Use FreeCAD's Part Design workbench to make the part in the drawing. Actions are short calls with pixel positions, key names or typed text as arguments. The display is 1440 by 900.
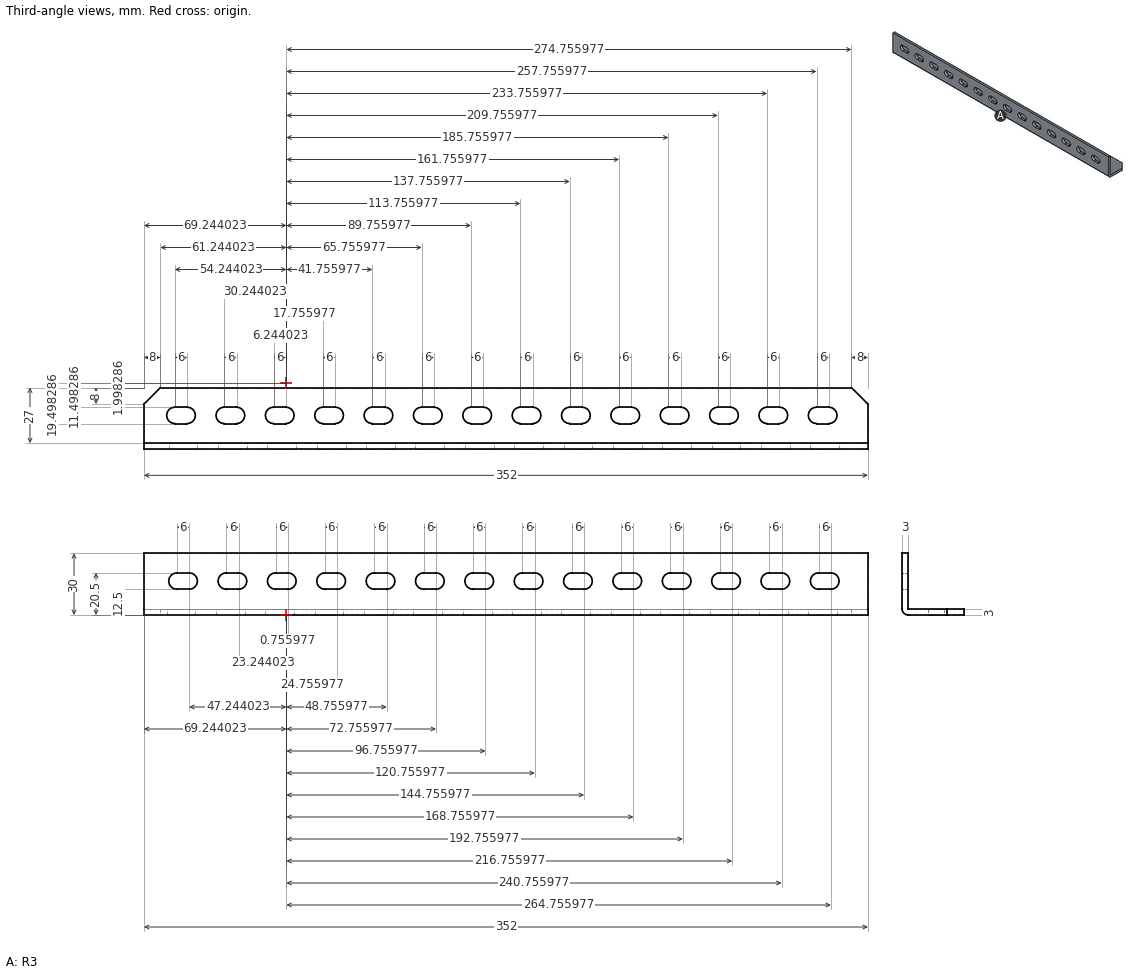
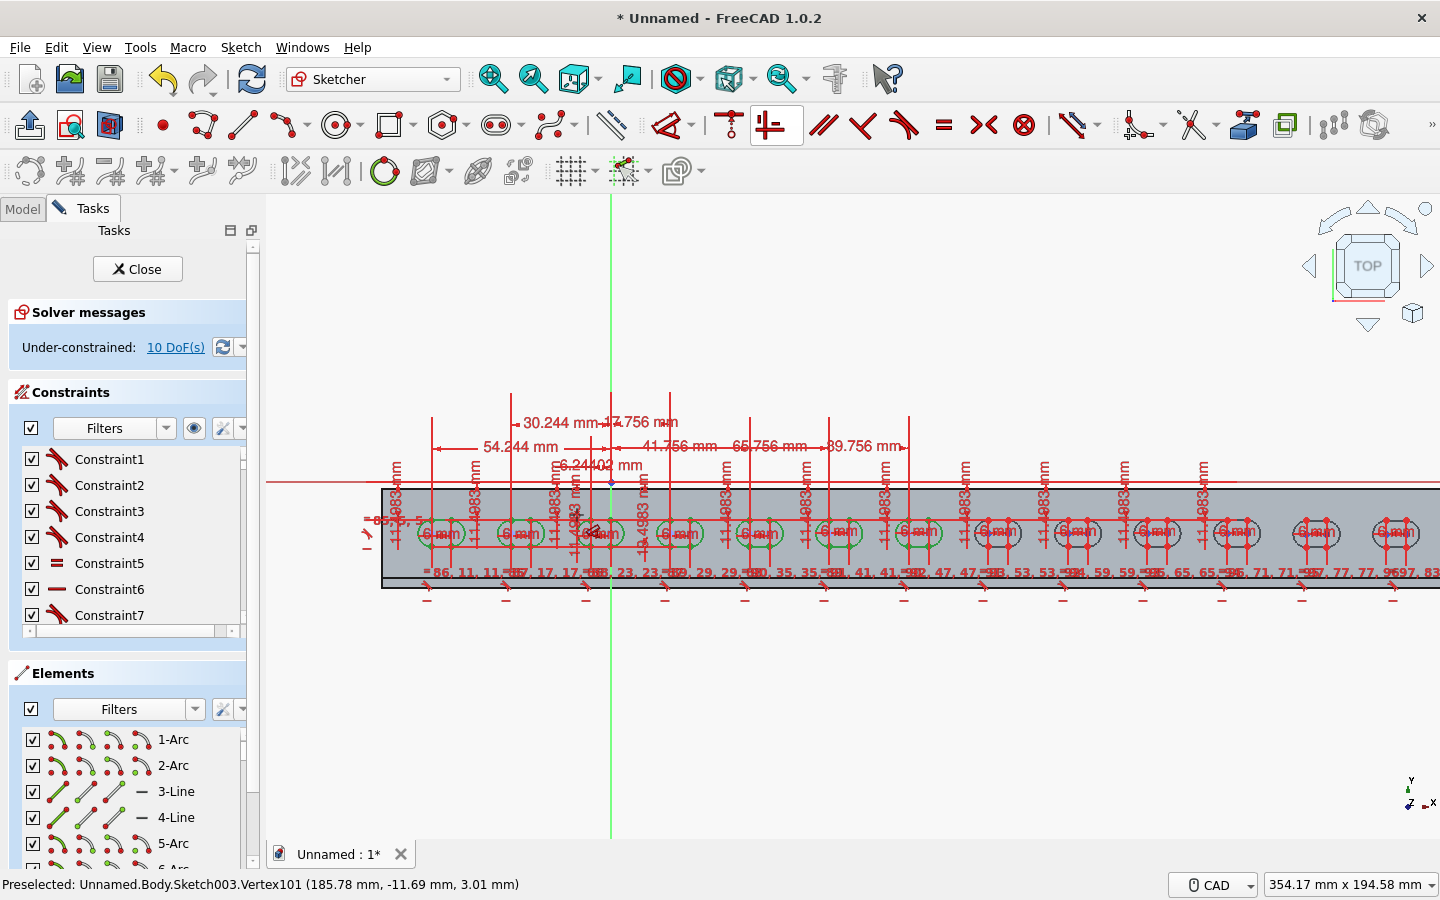
scroll(431, 521, down, 2)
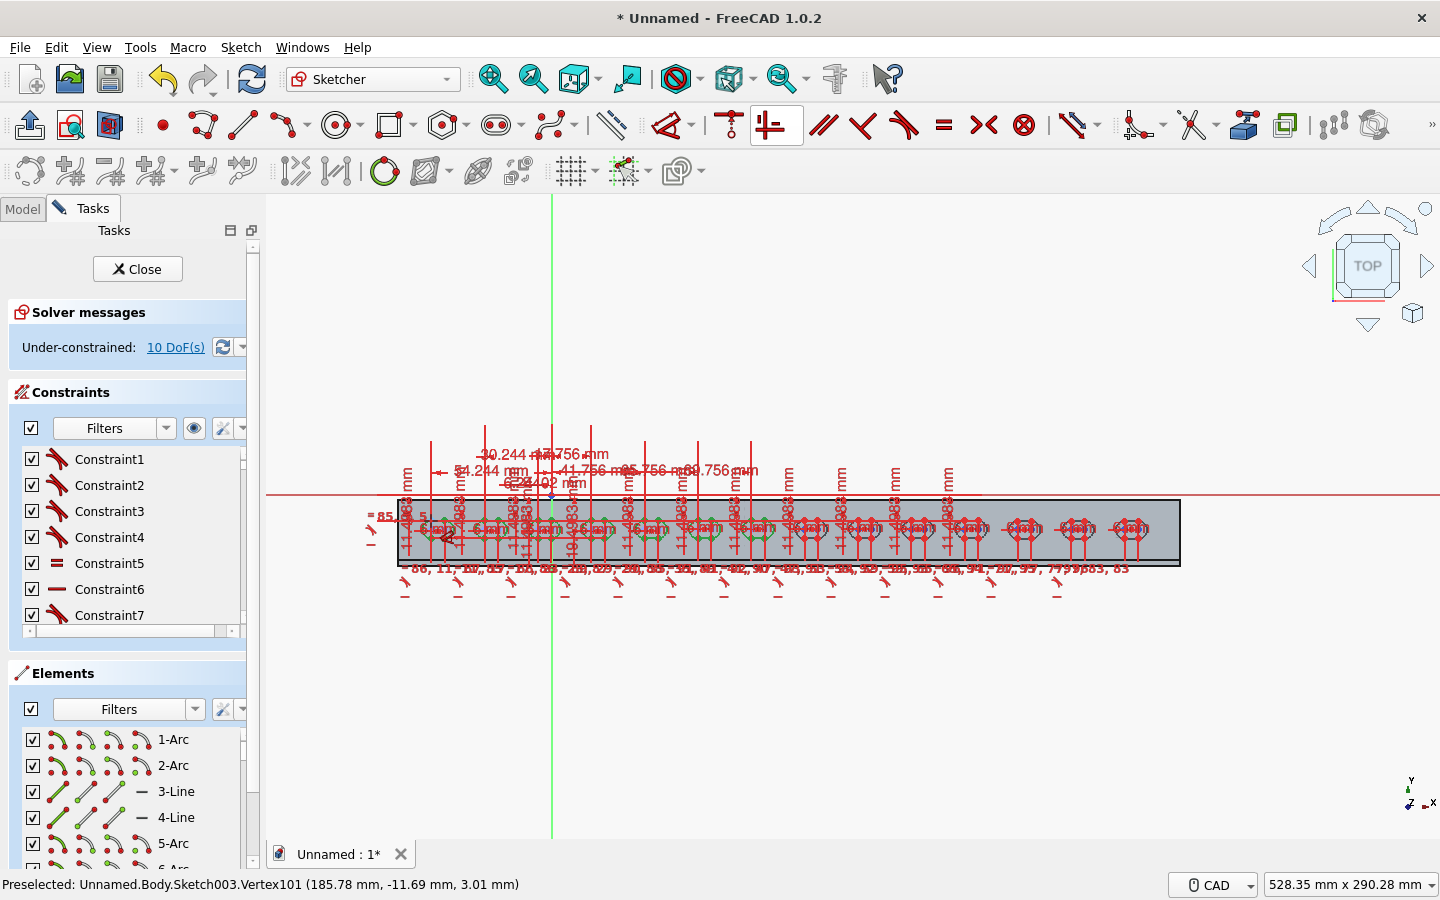
scroll(1018, 521, up, 3)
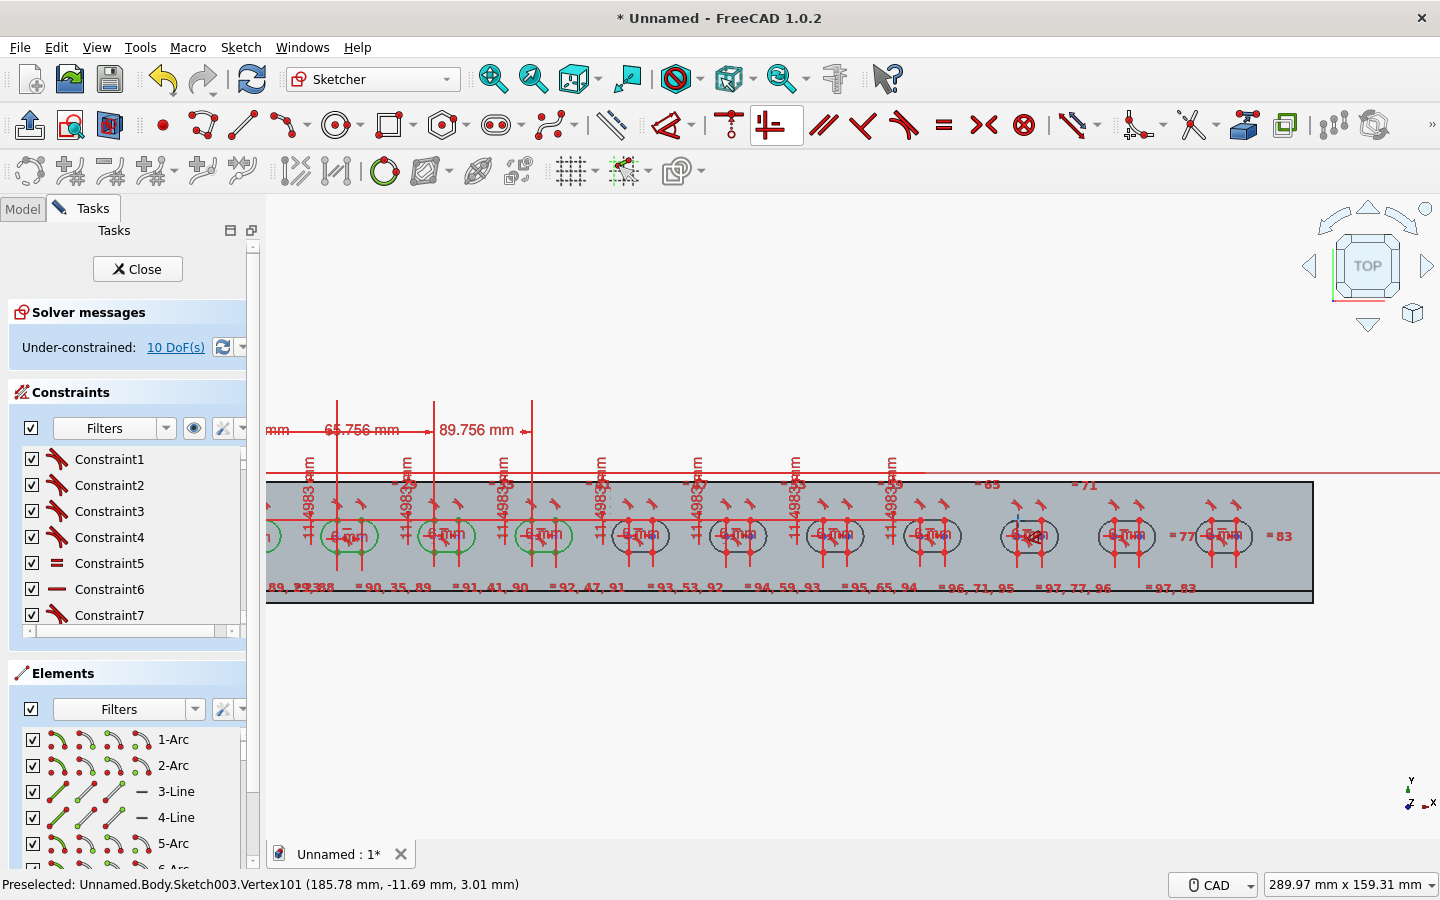
click(1017, 521)
click(1051, 497)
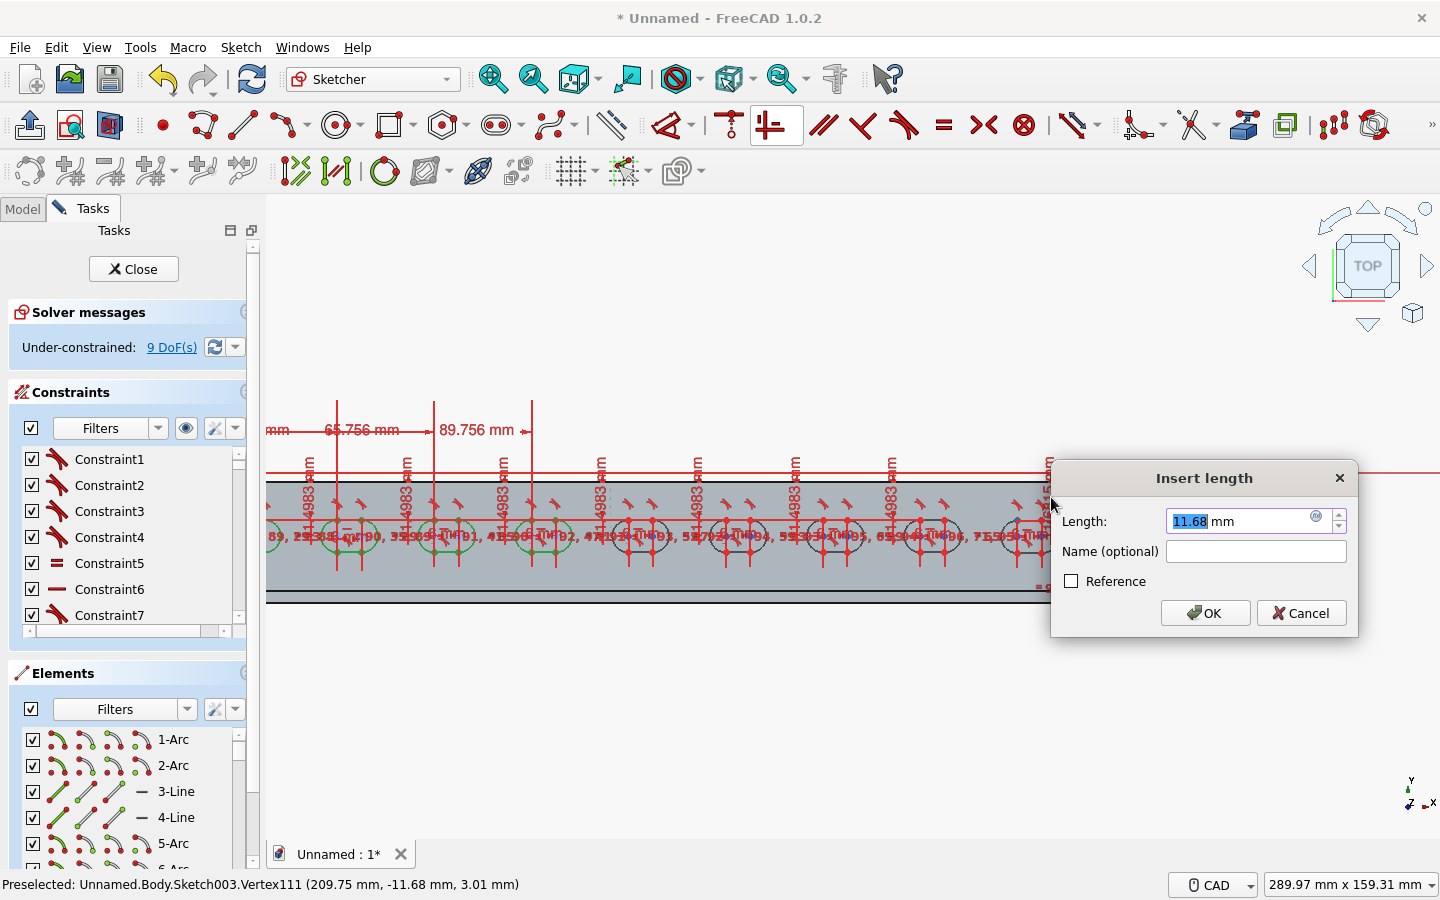
text(11.498286)
key(Return)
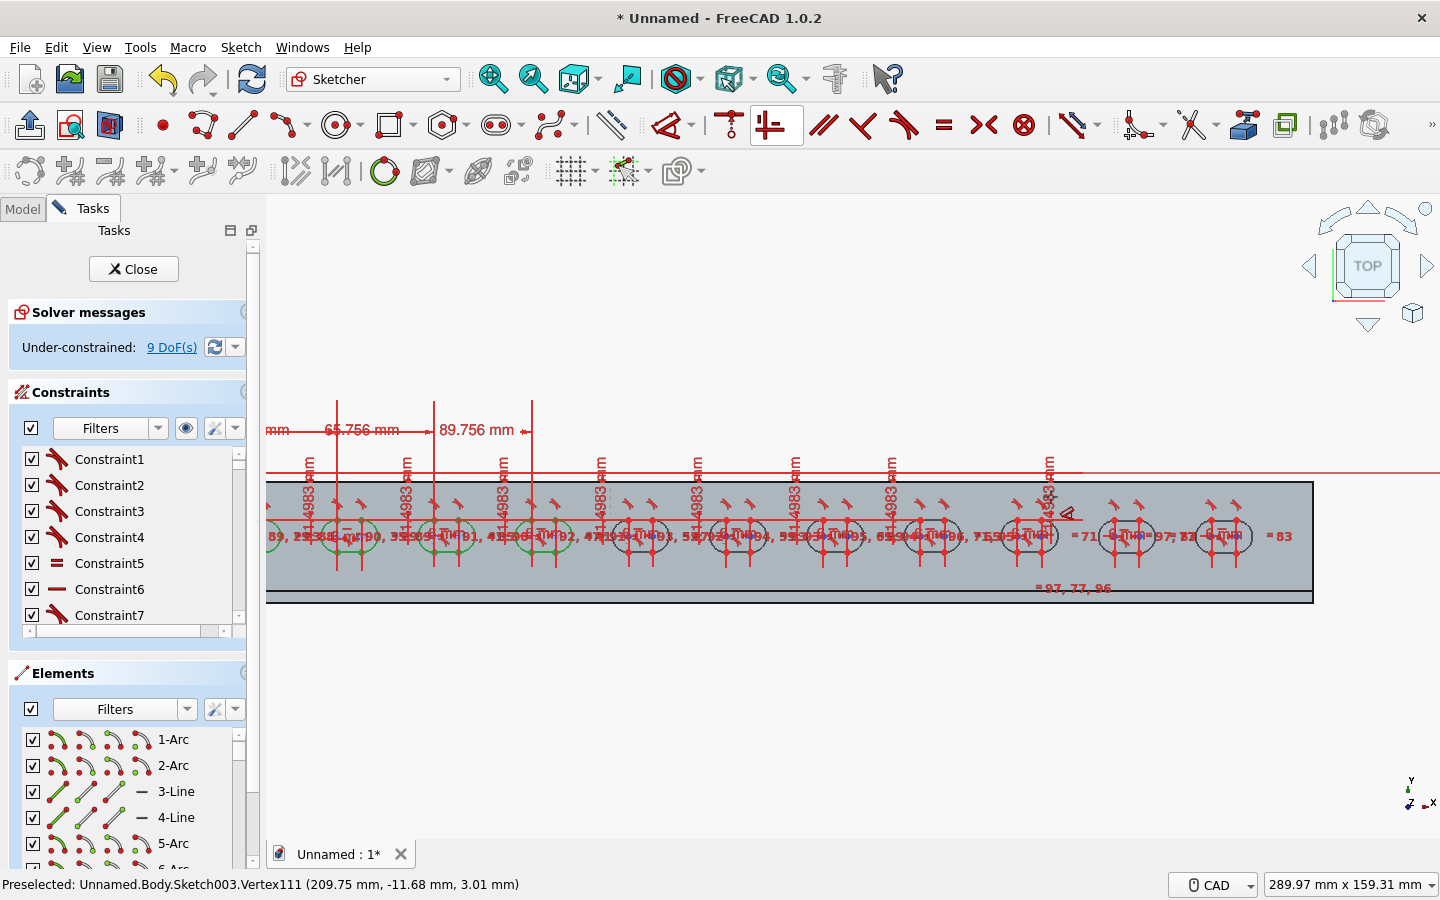
click(1115, 521)
click(1149, 497)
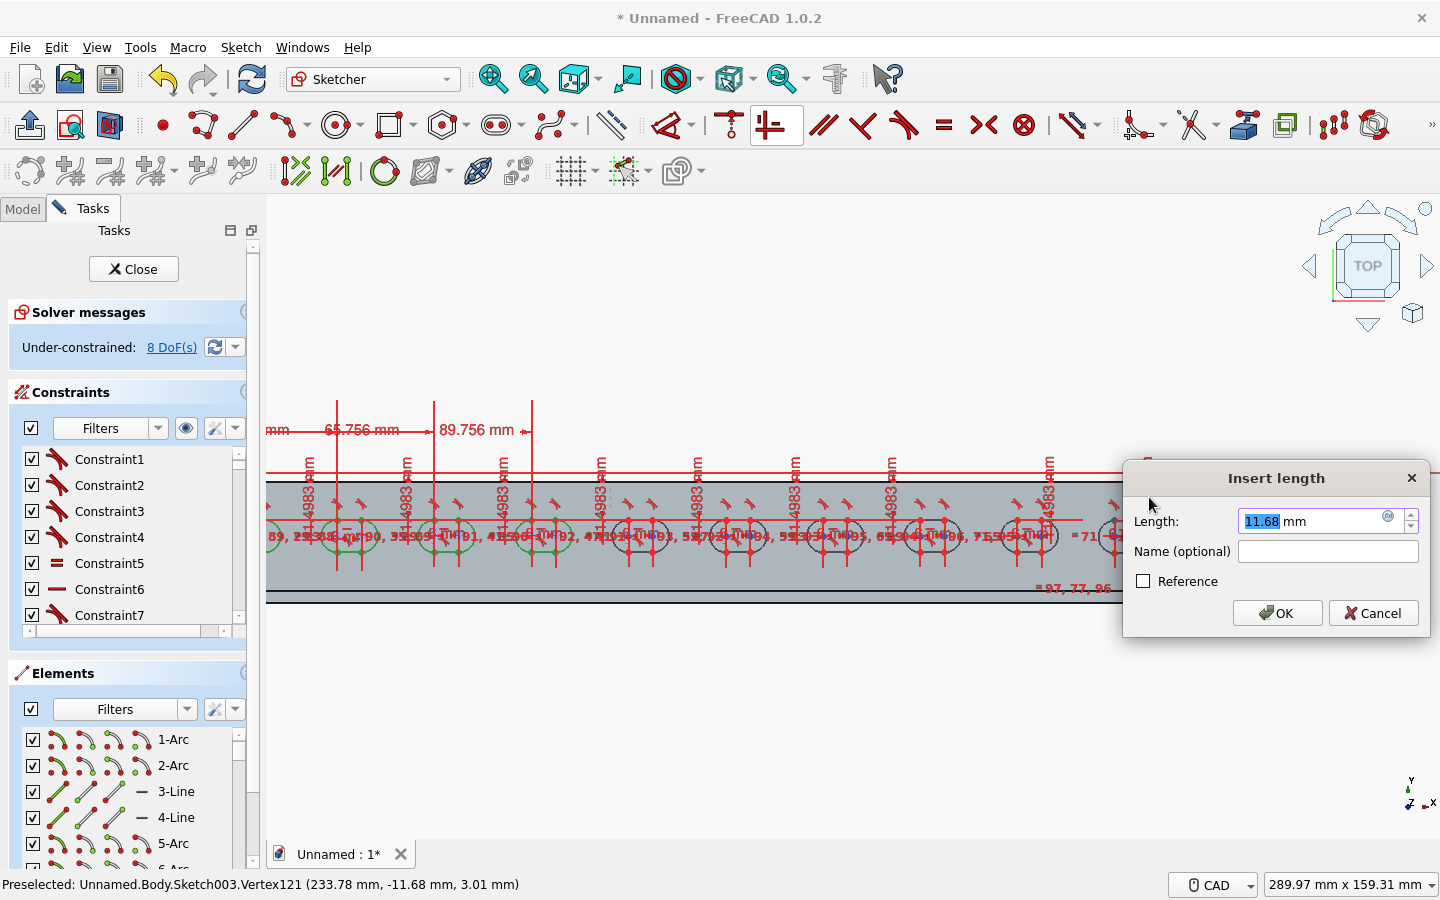
text(11.498286)
key(Return)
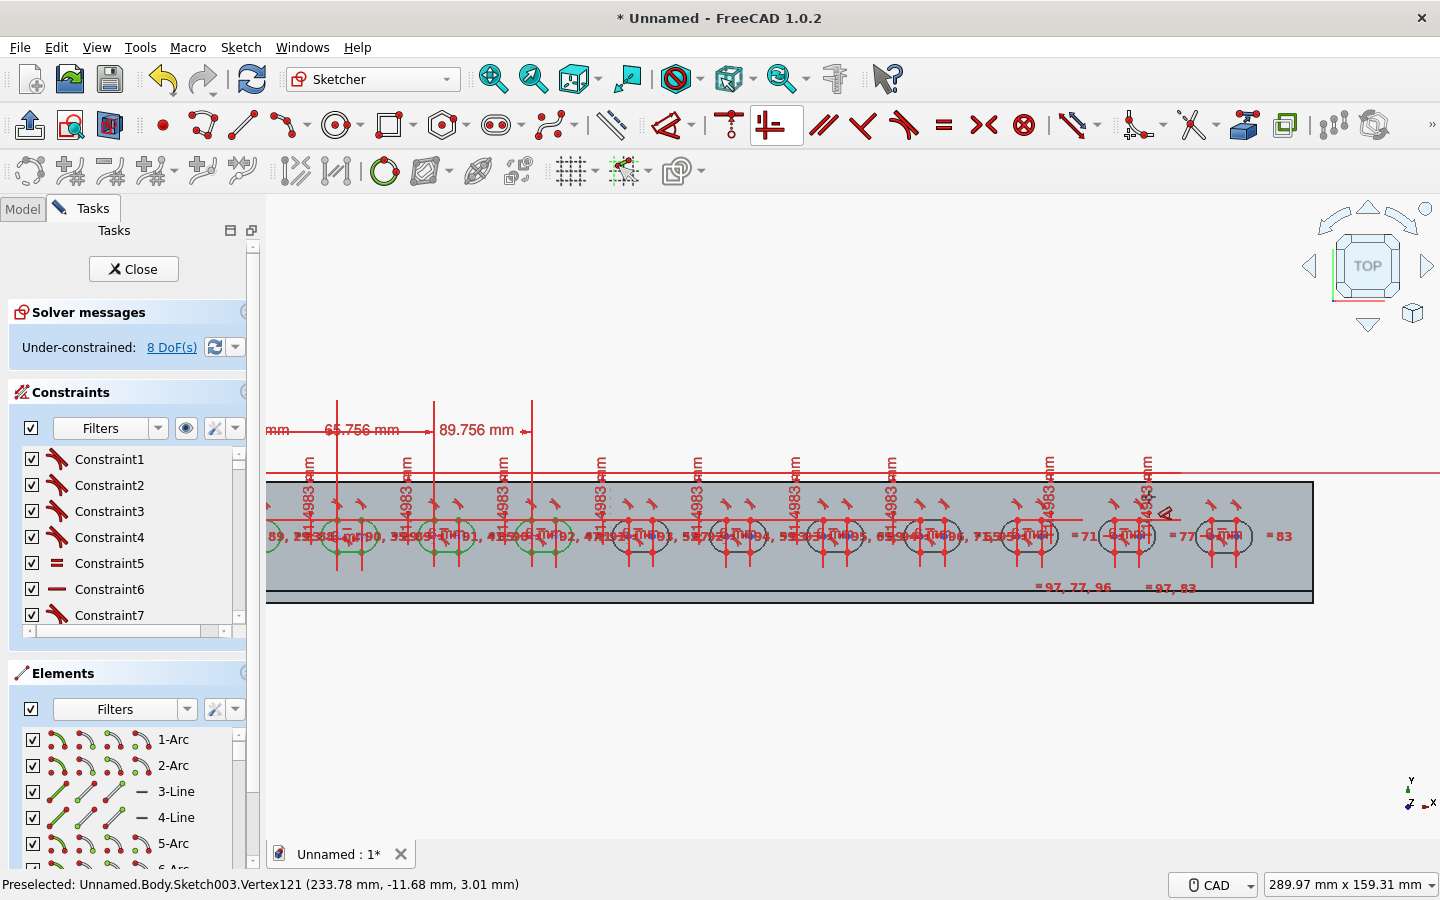
click(1212, 521)
click(1246, 497)